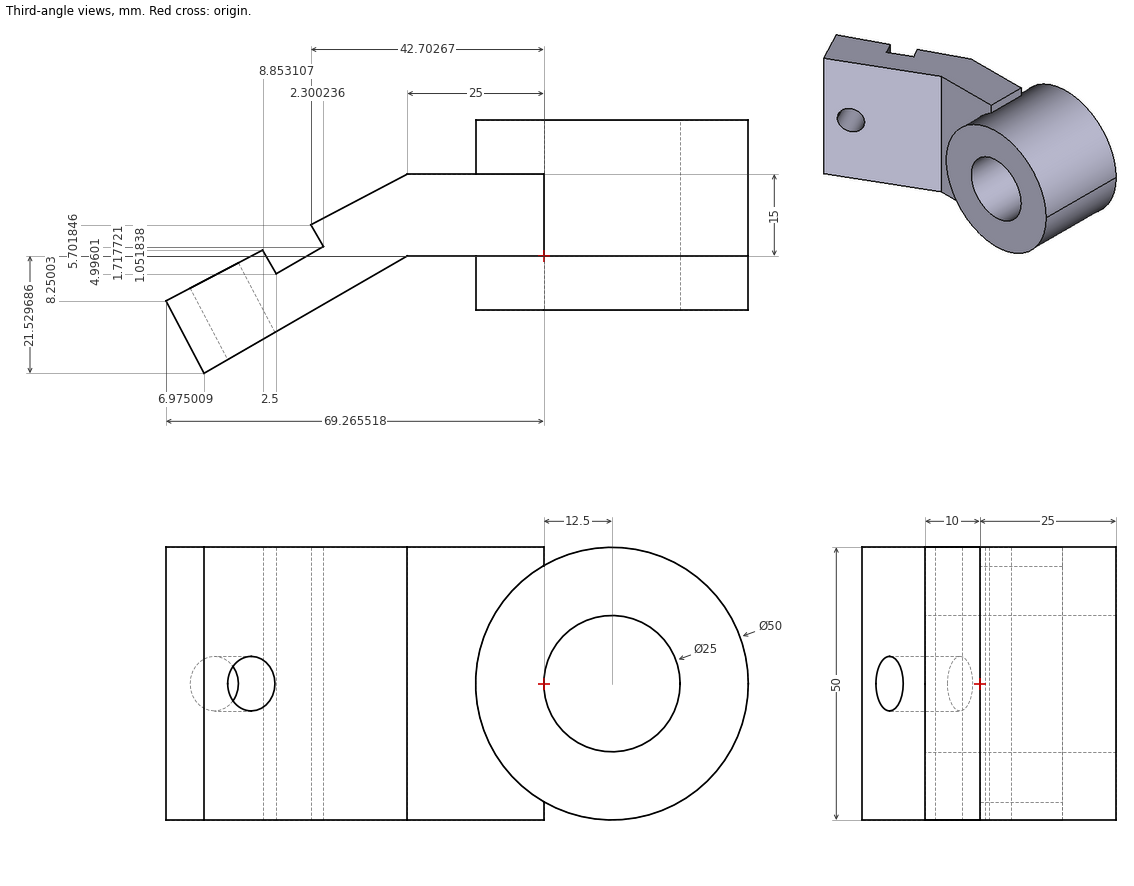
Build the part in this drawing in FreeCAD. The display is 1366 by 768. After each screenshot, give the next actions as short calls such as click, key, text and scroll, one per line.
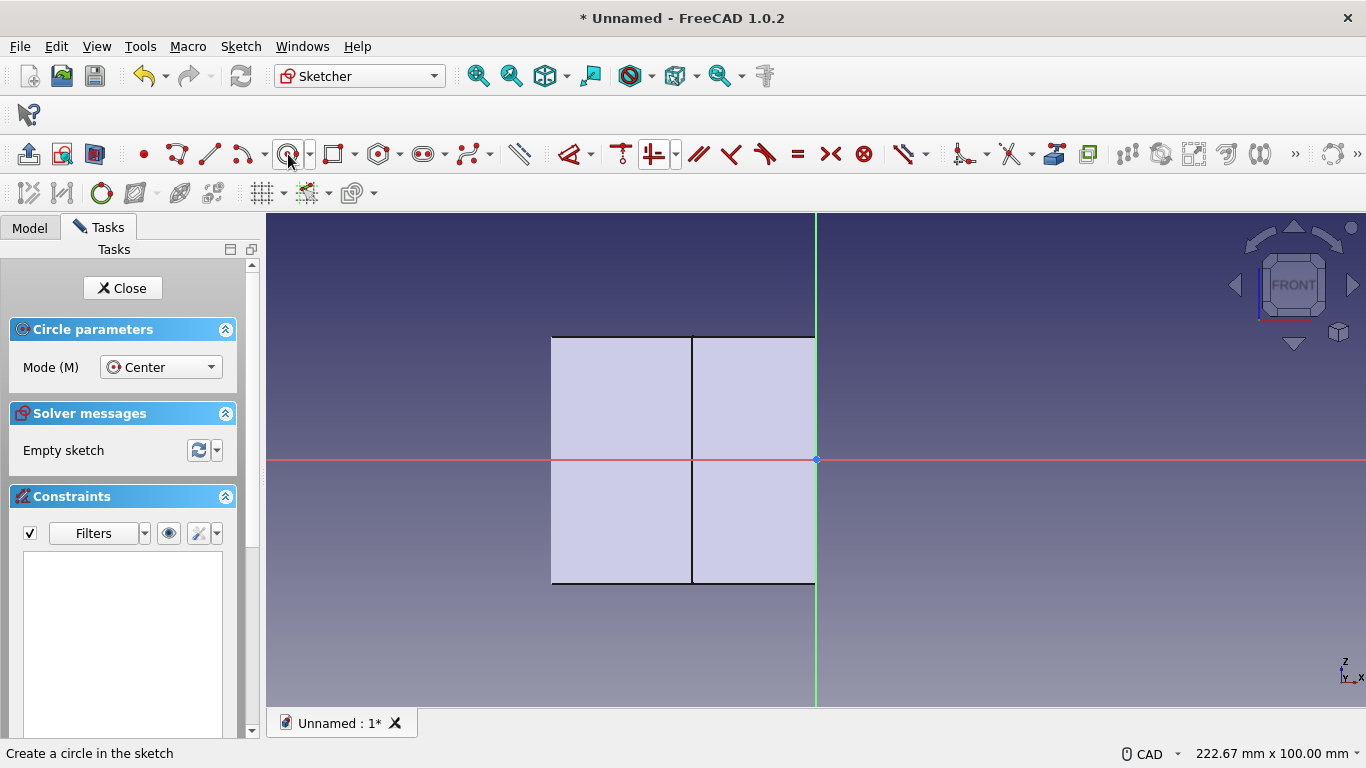
click(878, 460)
click(965, 373)
key(Escape)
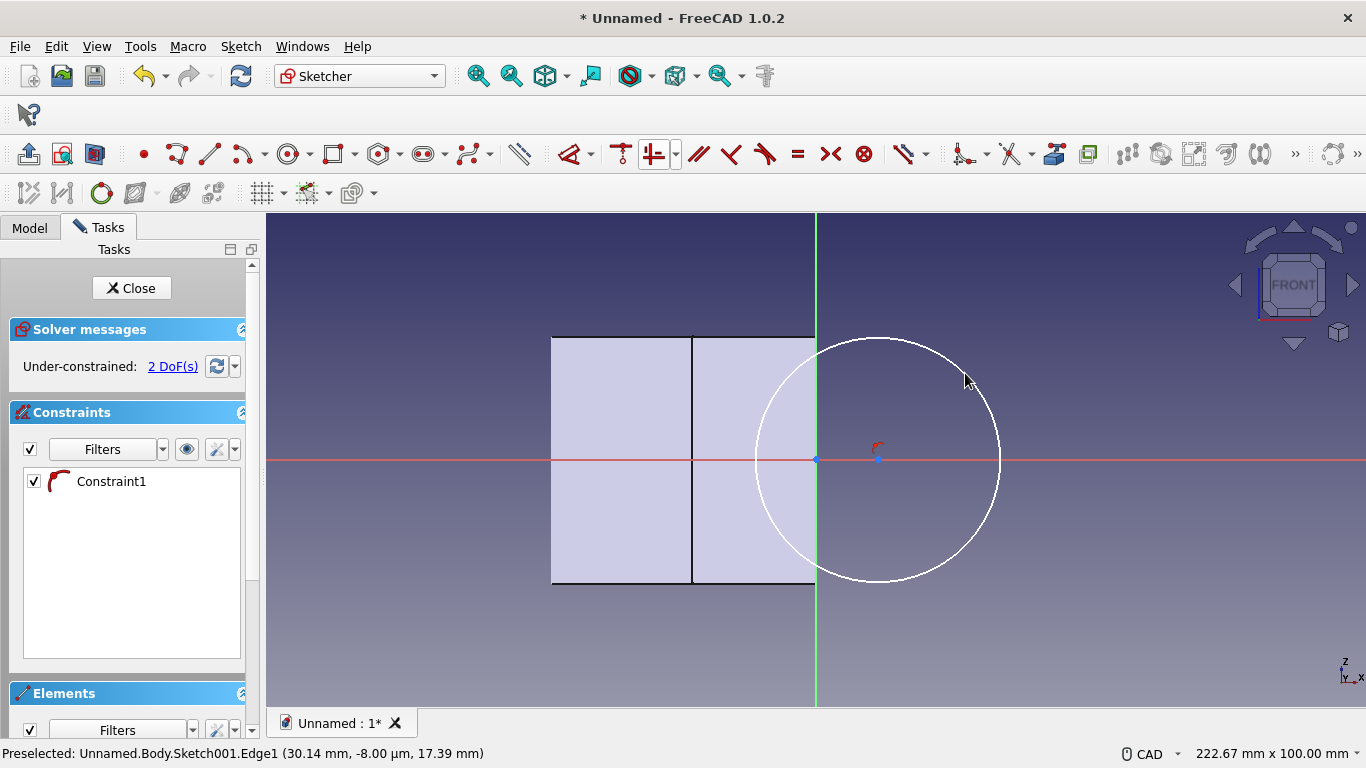
click(568, 154)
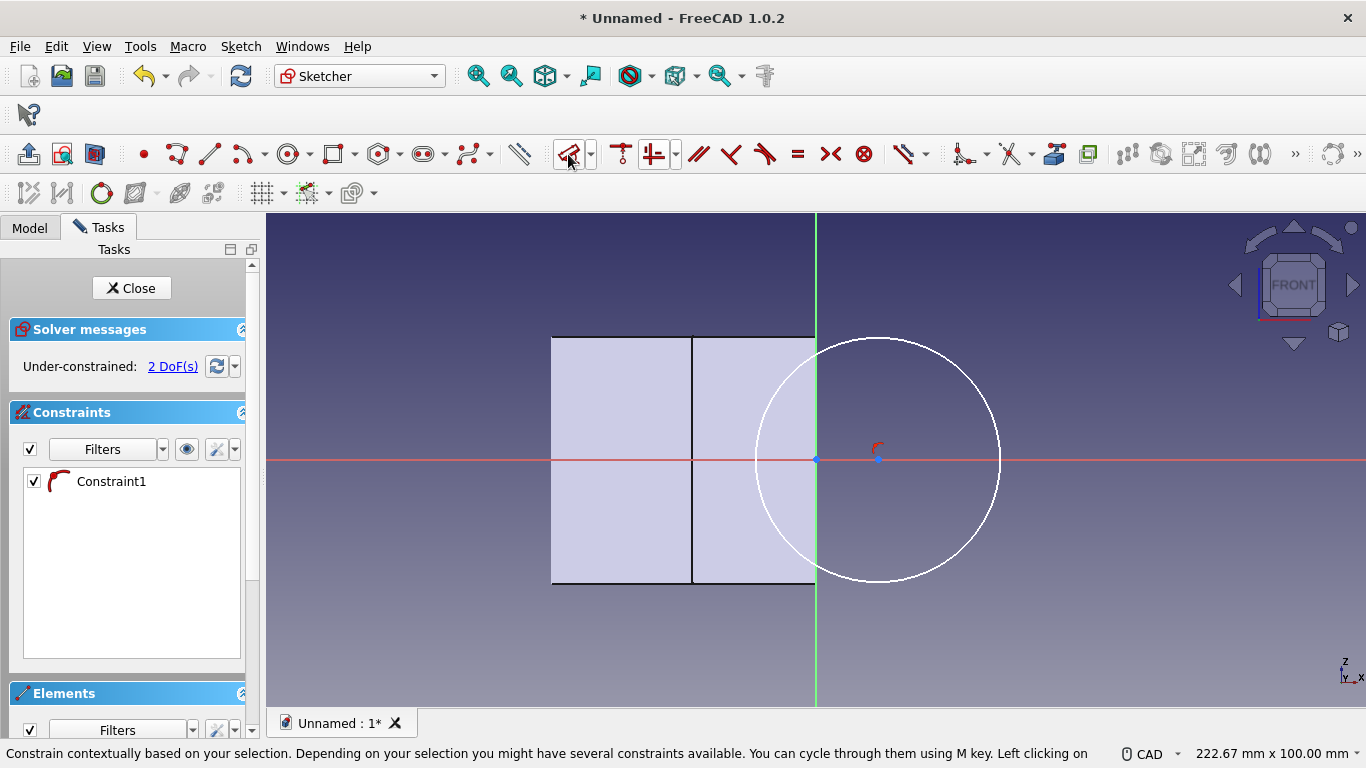
click(964, 373)
click(986, 350)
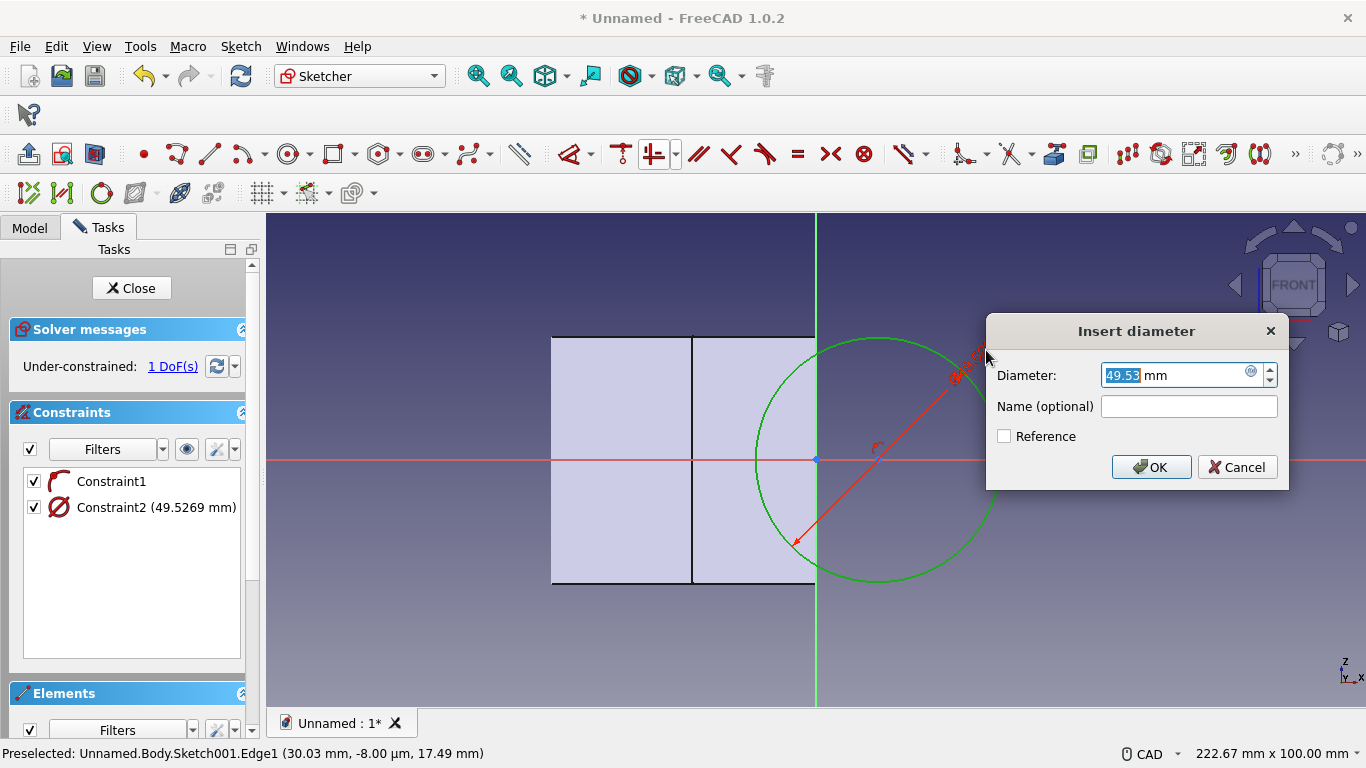
text(50)
key(Return)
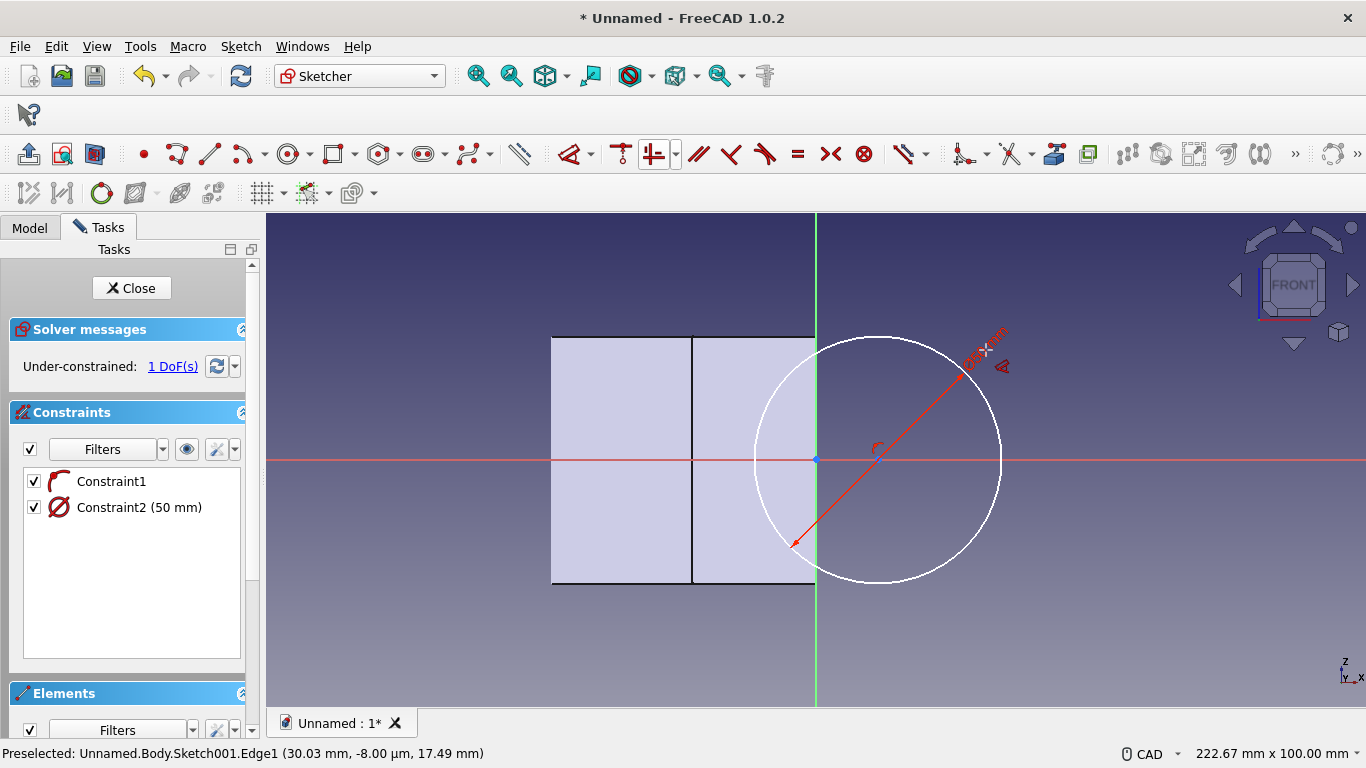
click(878, 460)
click(847, 494)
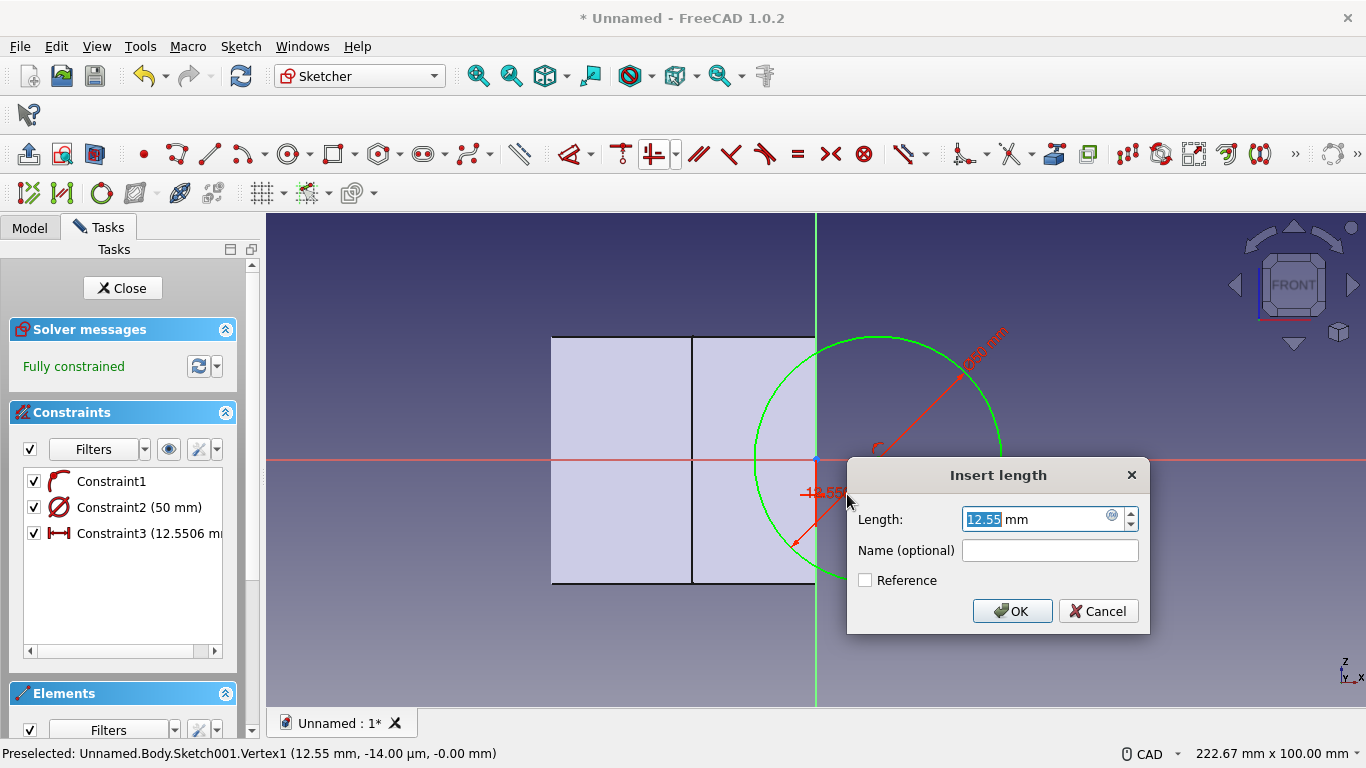
text(12.5)
key(Return)
key(Escape)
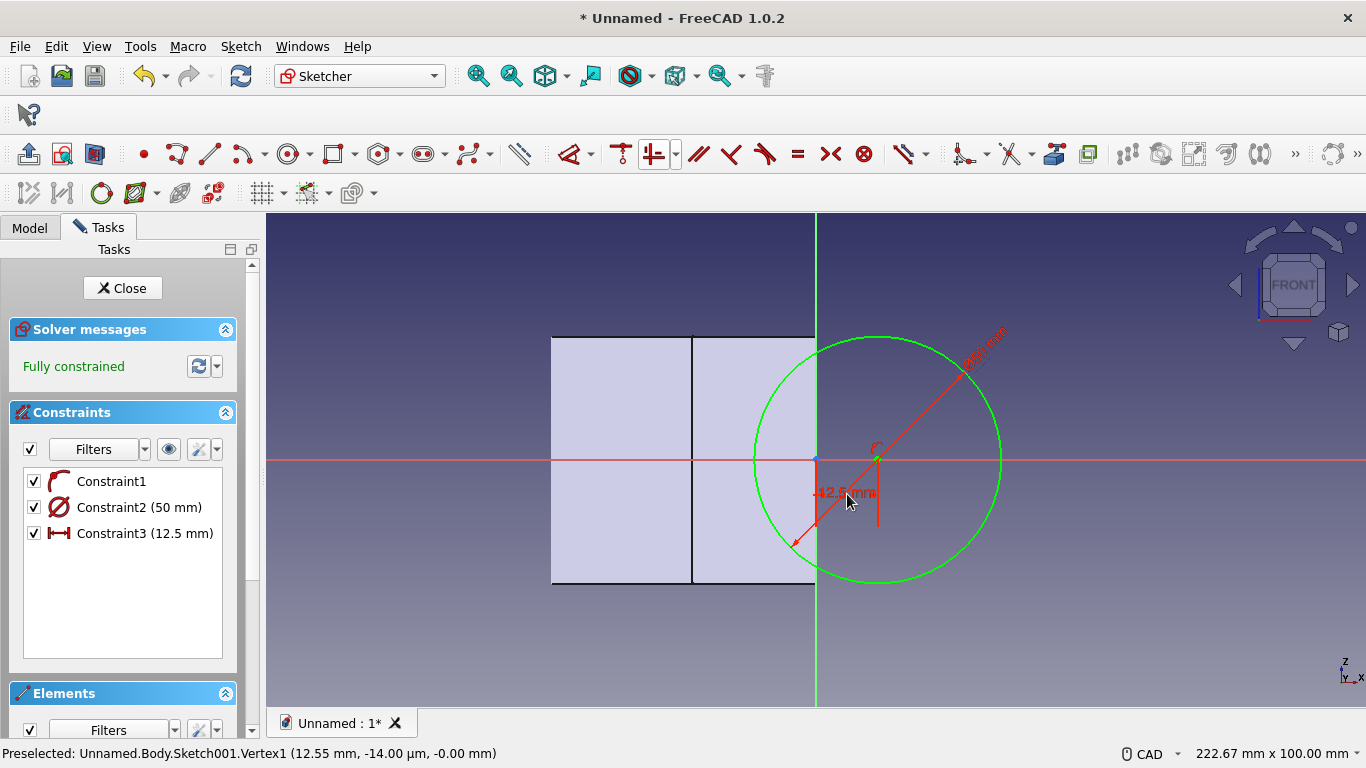
click(123, 288)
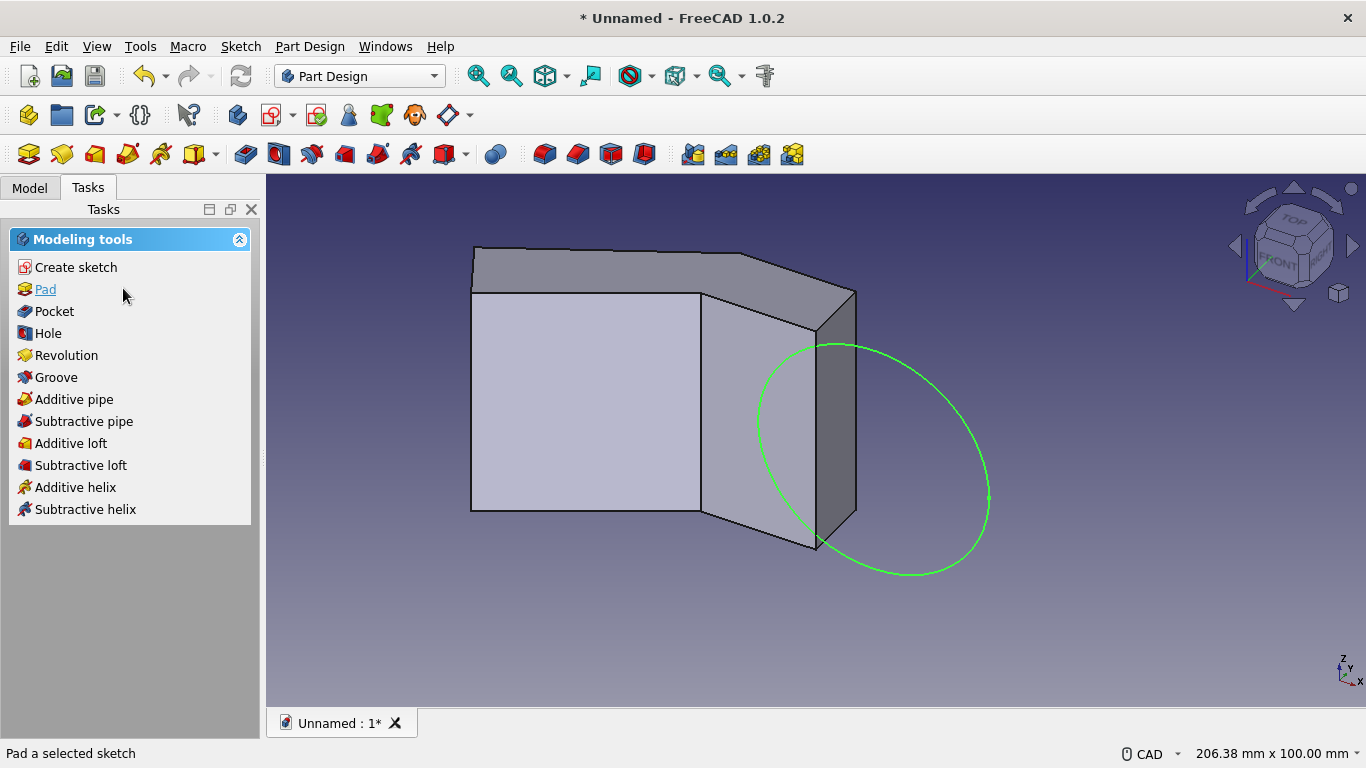
click(29, 154)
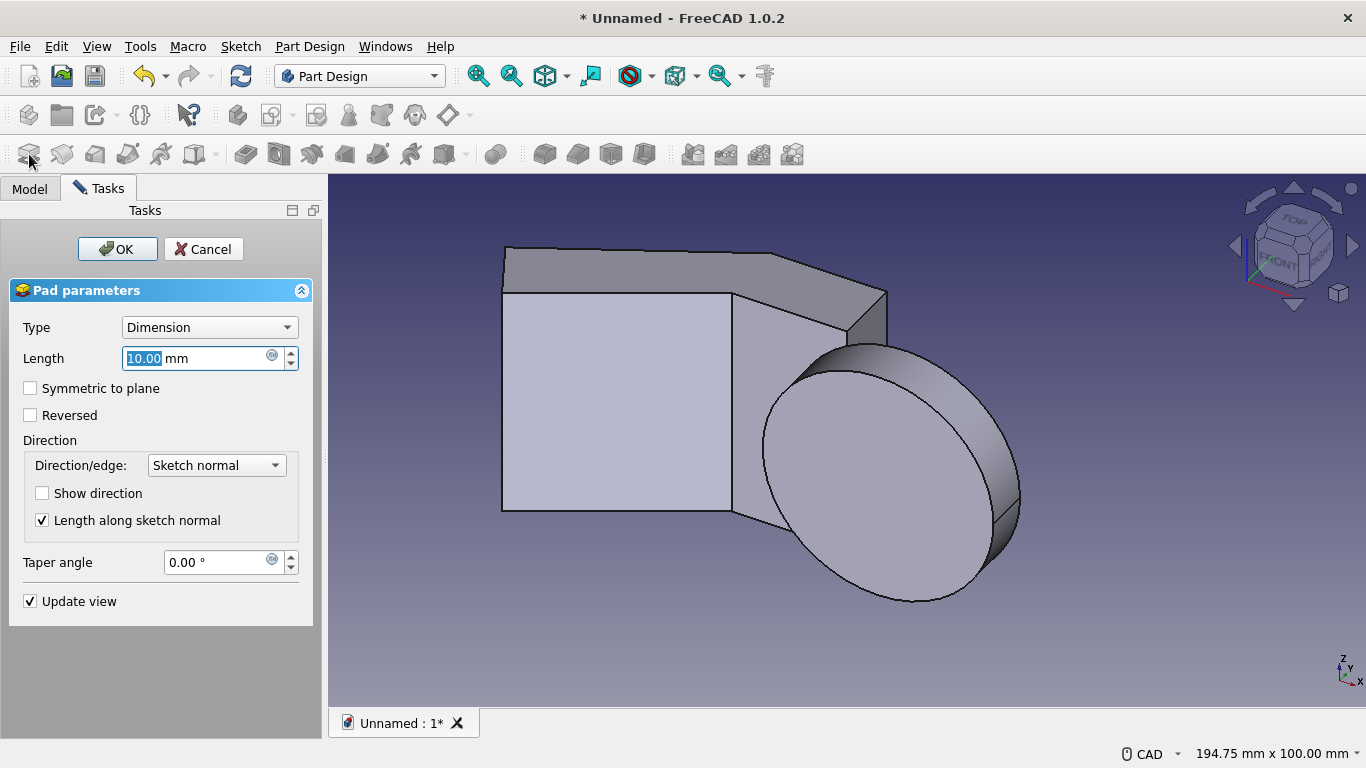
text(25)
key(Tab)